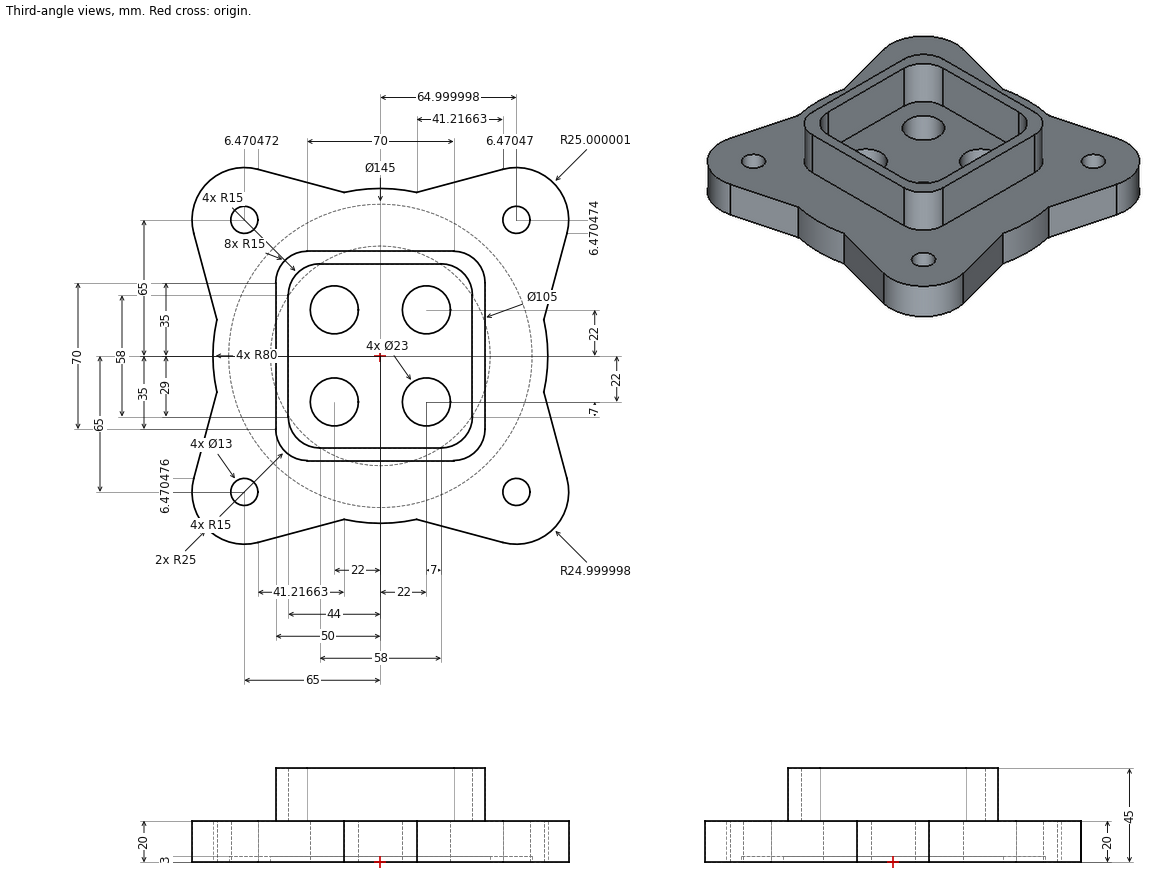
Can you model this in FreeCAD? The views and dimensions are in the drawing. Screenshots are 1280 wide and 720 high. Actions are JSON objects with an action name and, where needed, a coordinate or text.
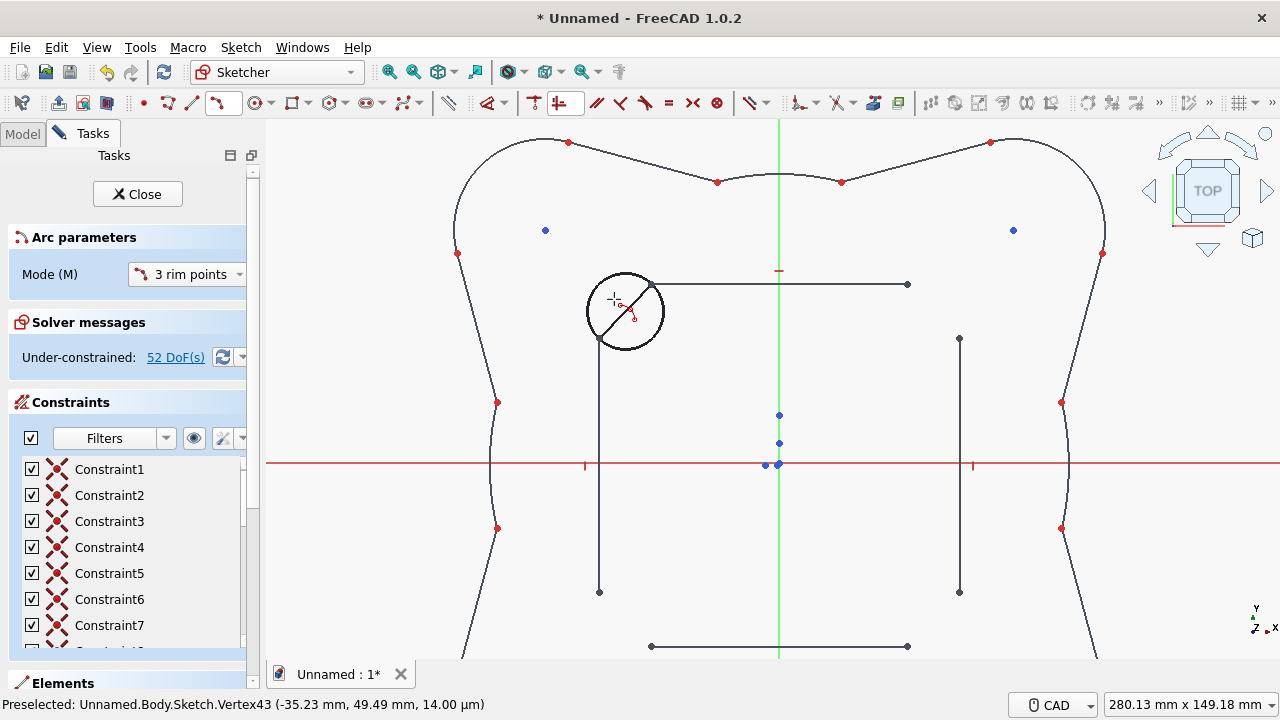
{"action": "left_click", "coordinate": [614, 298]}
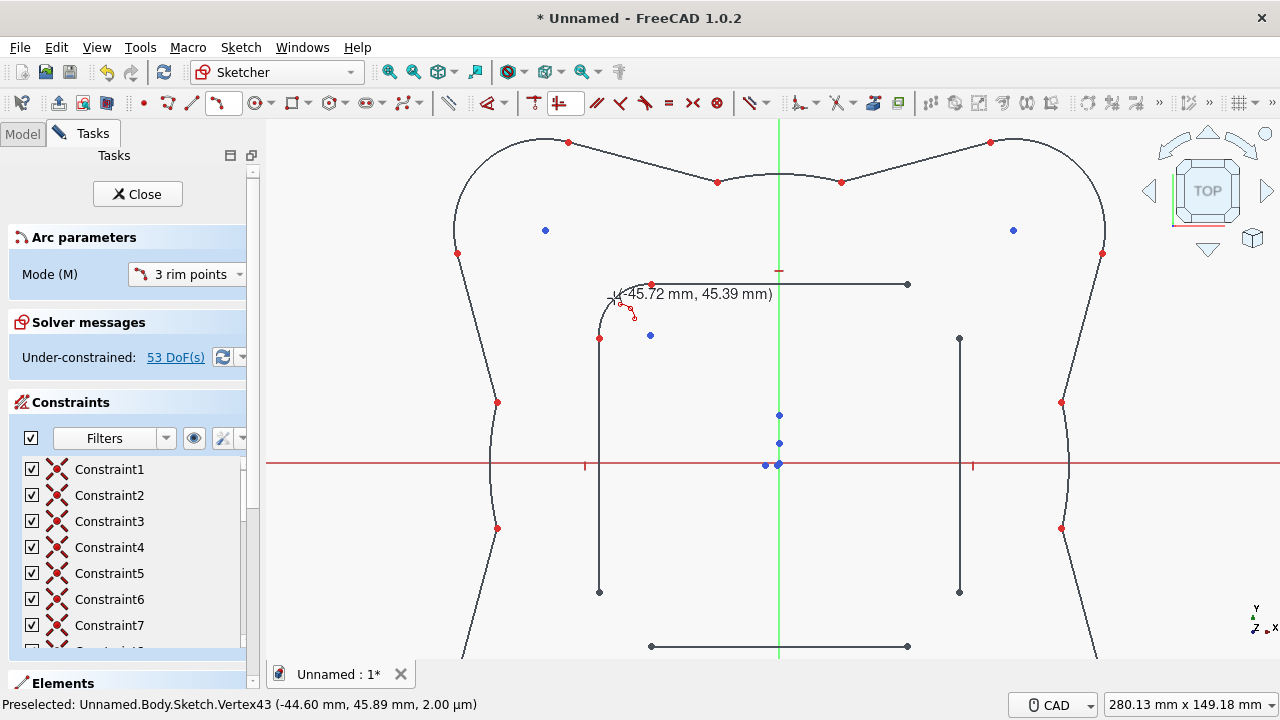
{"action": "left_click", "coordinate": [907, 284]}
{"action": "left_click", "coordinate": [960, 339]}
{"action": "left_click", "coordinate": [945, 298]}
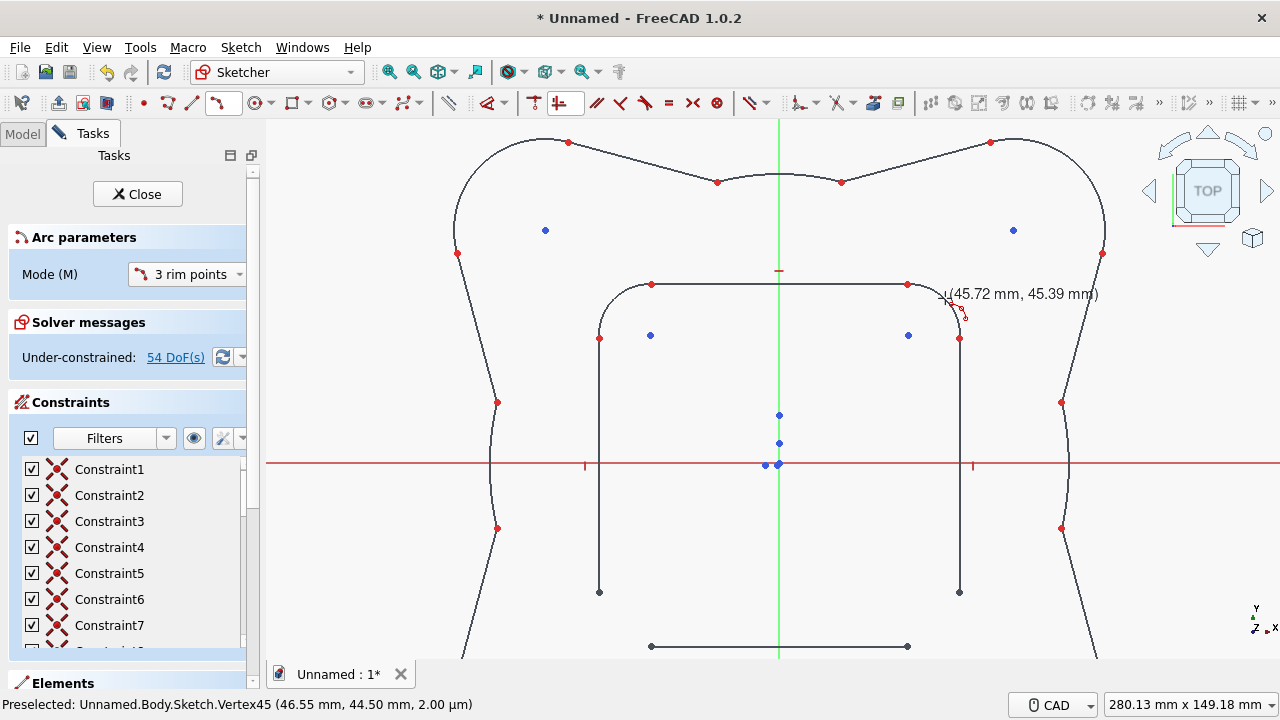
{"action": "left_click", "coordinate": [960, 592]}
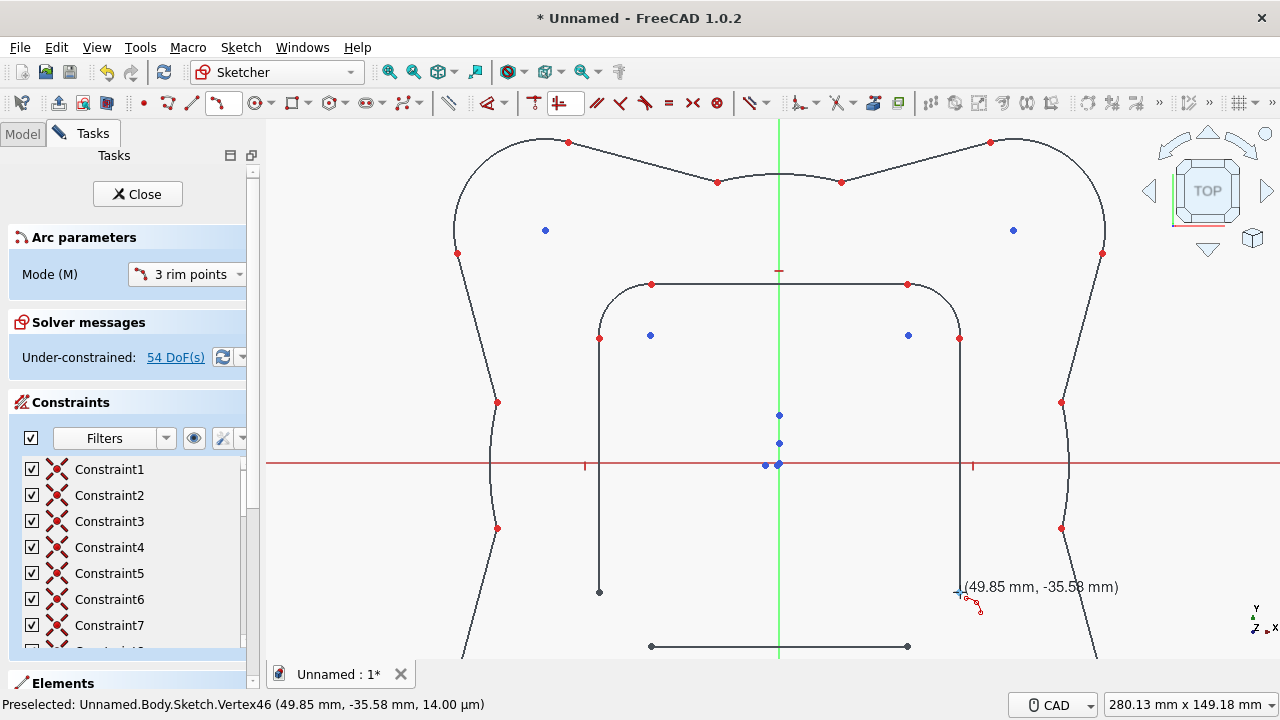
{"action": "scroll", "coordinate": [613, 299], "scroll_direction": "down", "scroll_amount": 3}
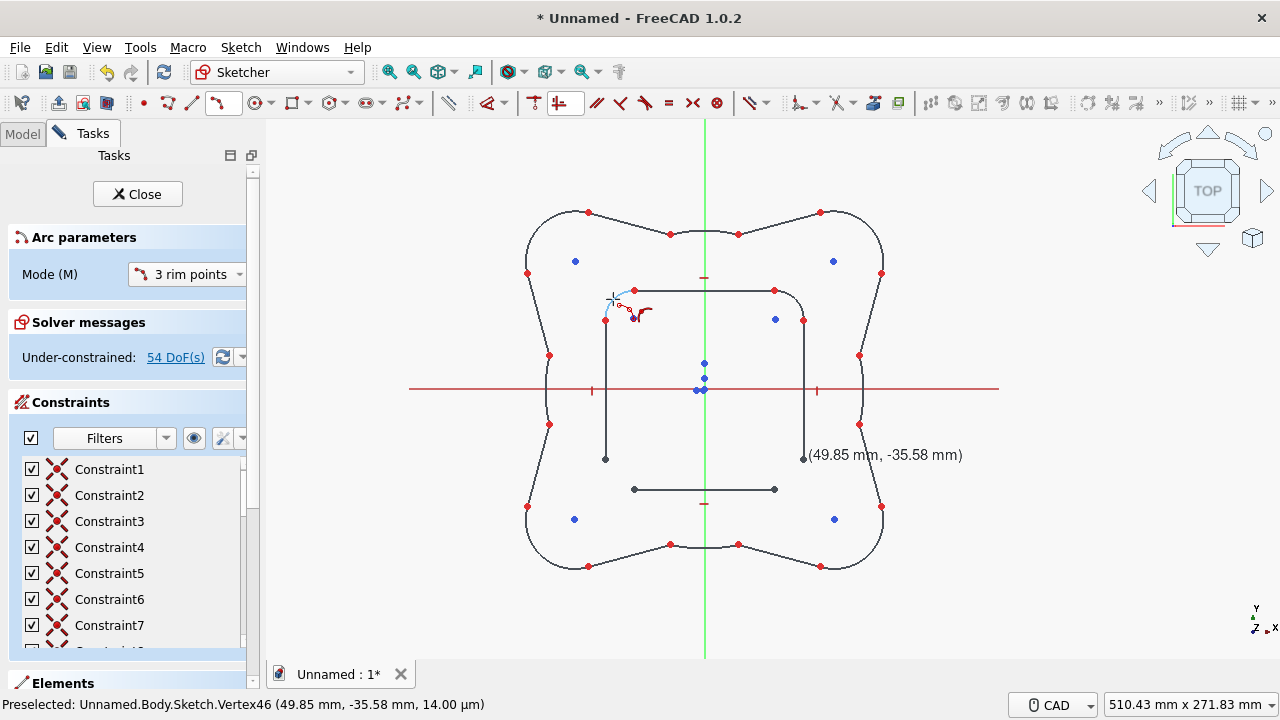
{"action": "left_click", "coordinate": [775, 490]}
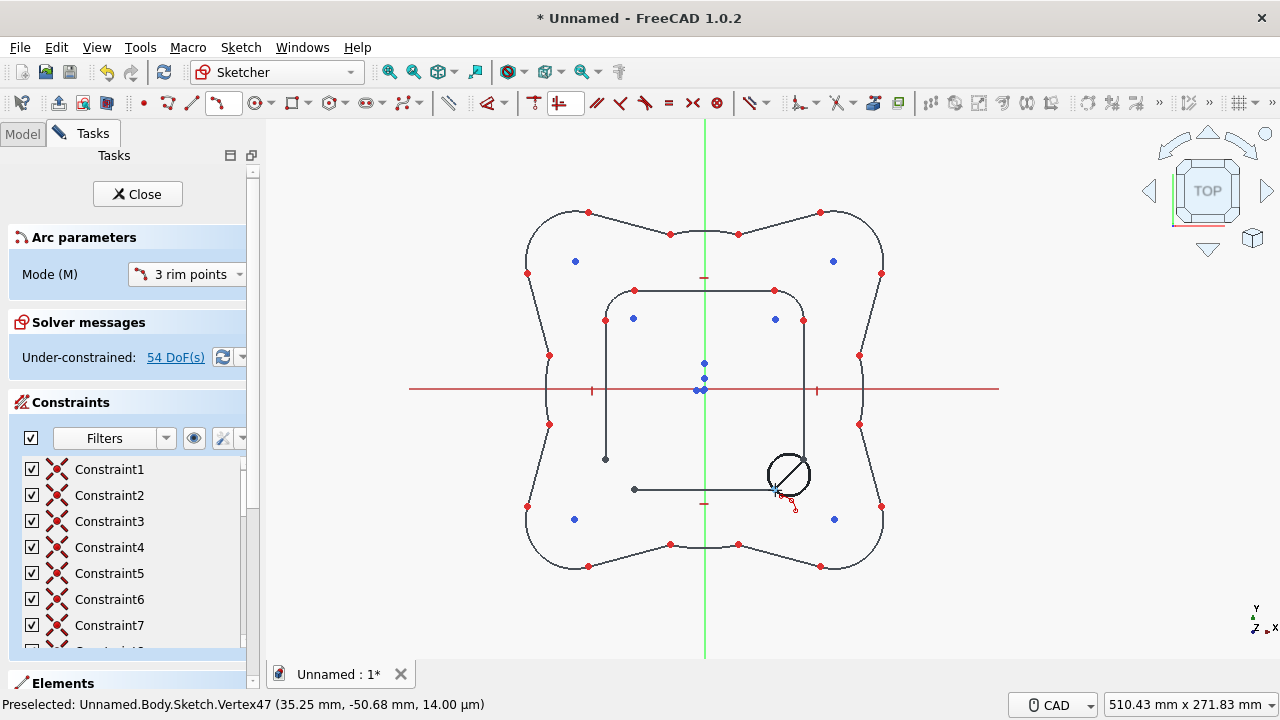
{"action": "scroll", "coordinate": [795, 480], "scroll_direction": "up", "scroll_amount": 3}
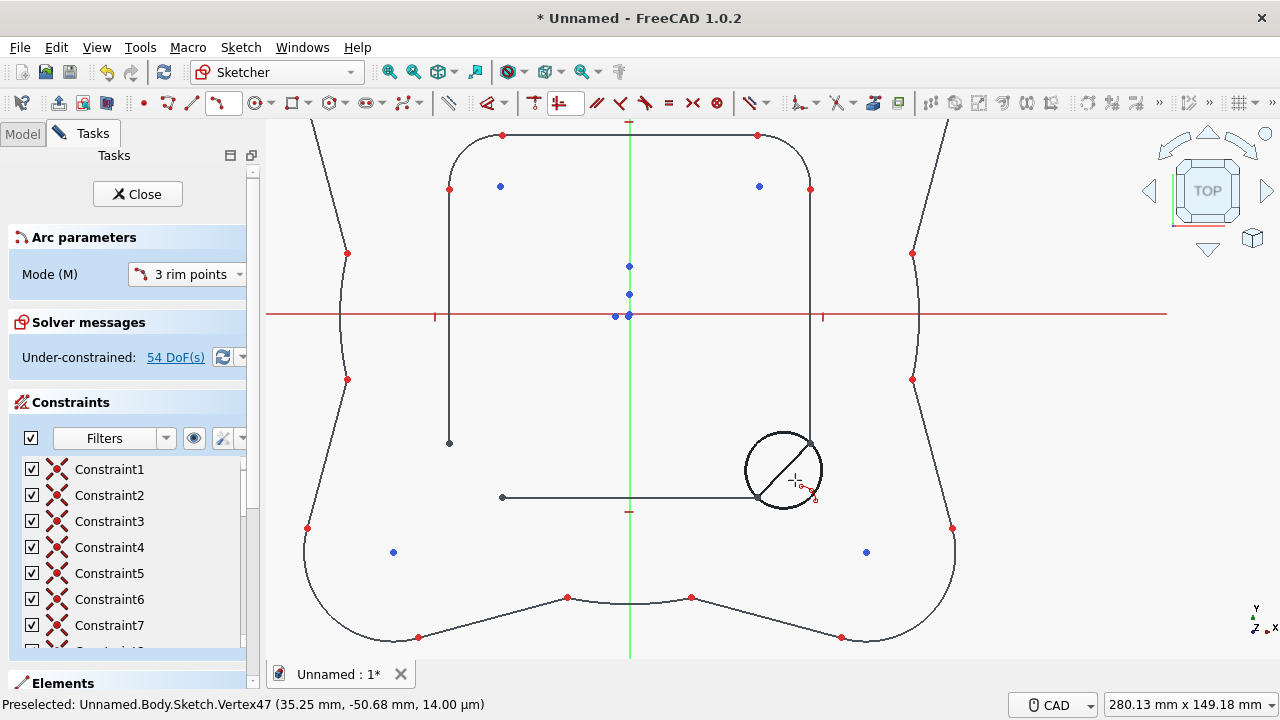
{"action": "left_click", "coordinate": [795, 479]}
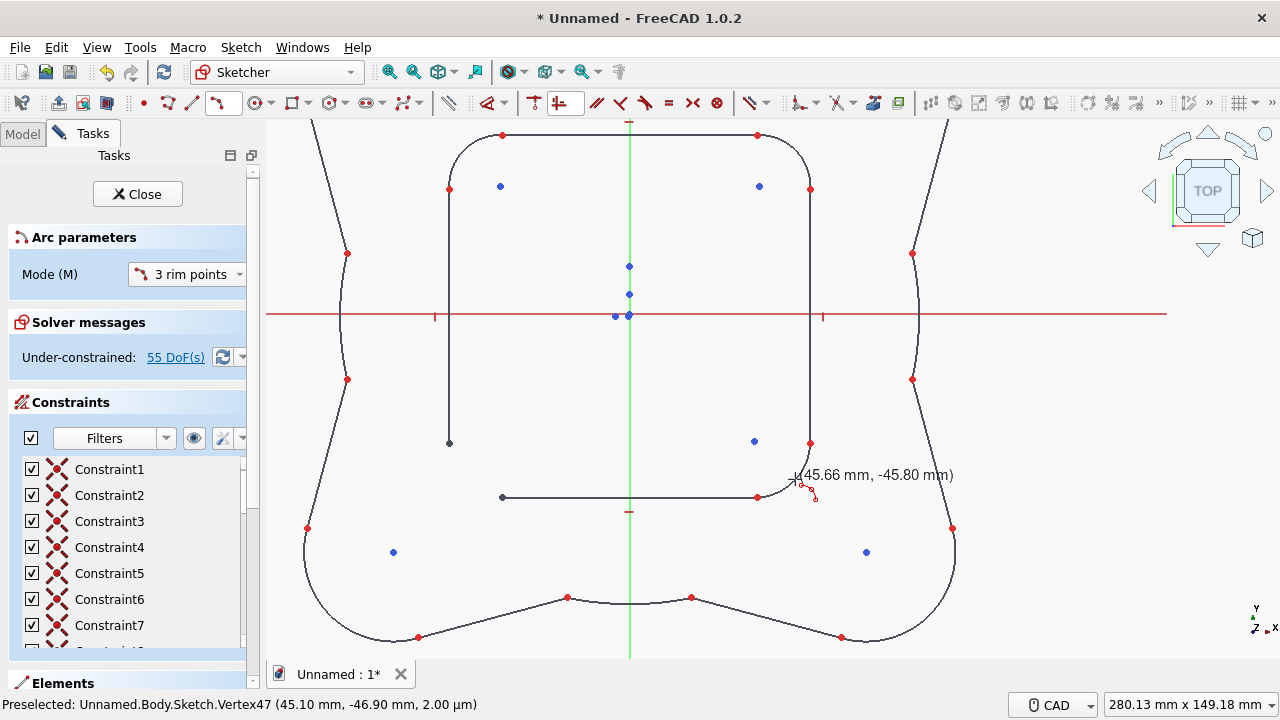
{"action": "left_click", "coordinate": [502, 498]}
{"action": "left_click", "coordinate": [449, 443]}
{"action": "left_click", "coordinate": [465, 479]}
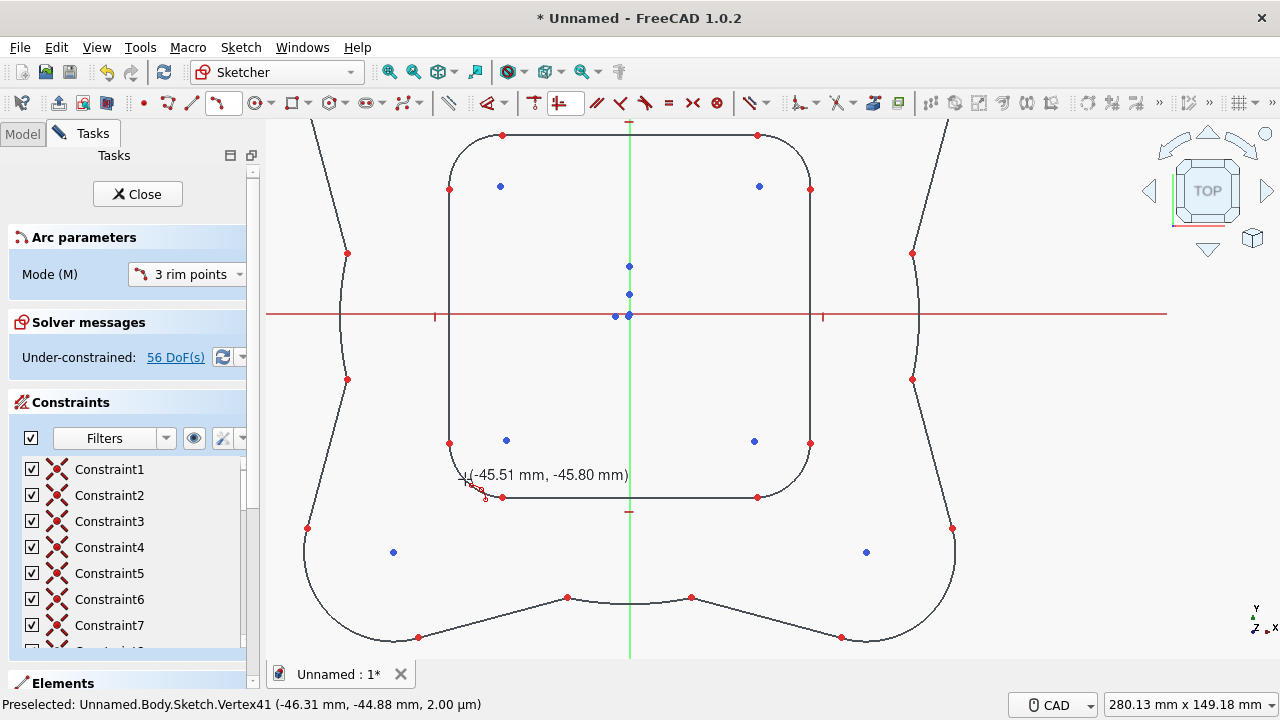
{"action": "key", "text": "g c"}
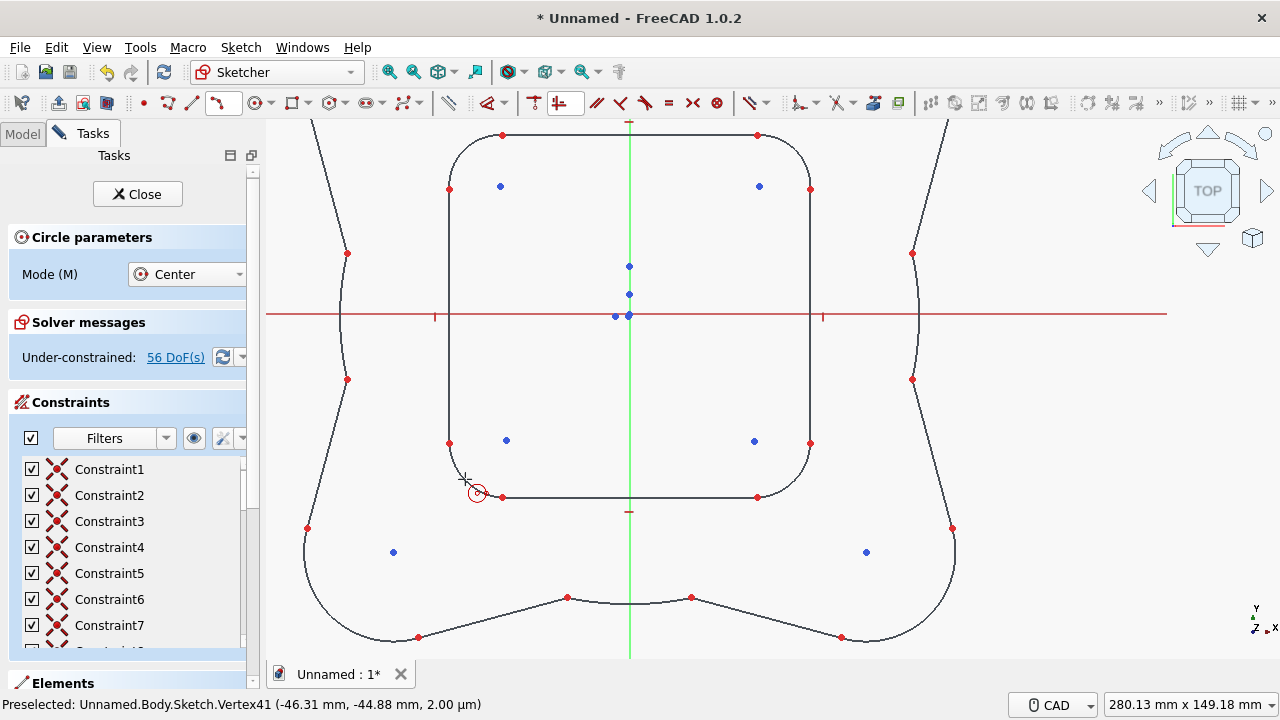
{"action": "left_click", "coordinate": [394, 549]}
{"action": "mouse_move", "coordinate": [411, 533]}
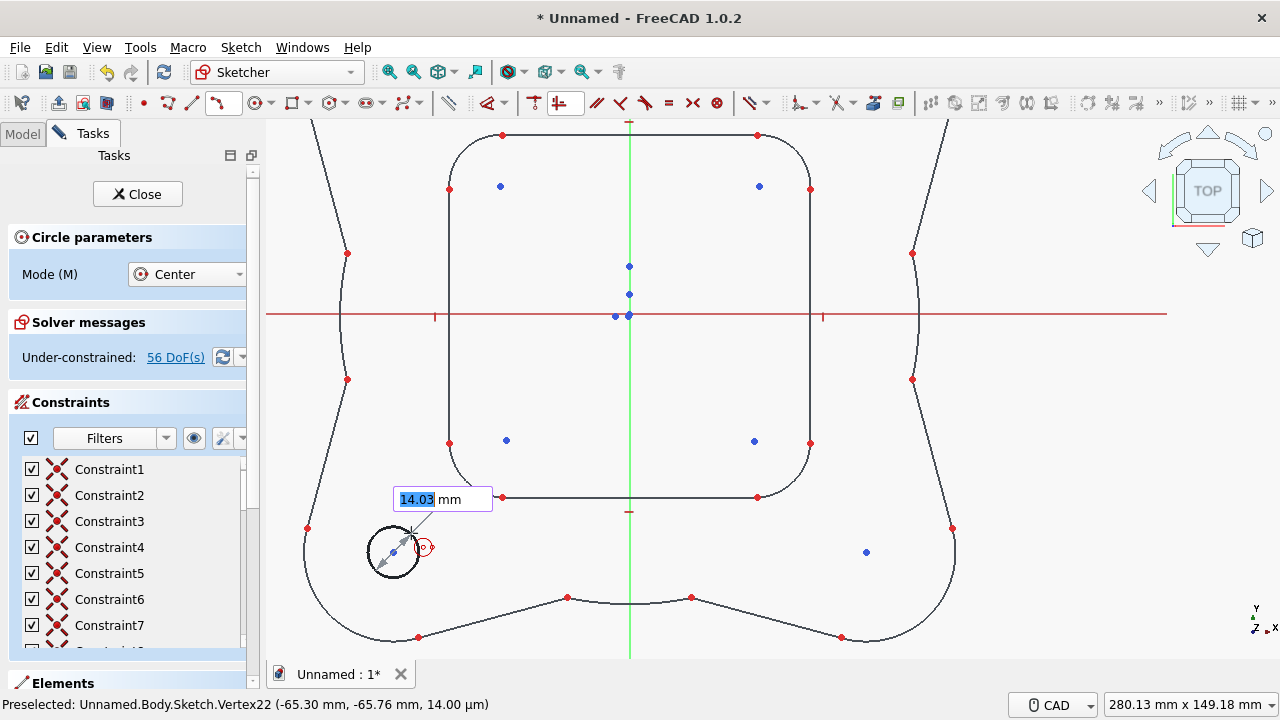
{"action": "type", "text": "13"}
{"action": "key", "text": "Return"}